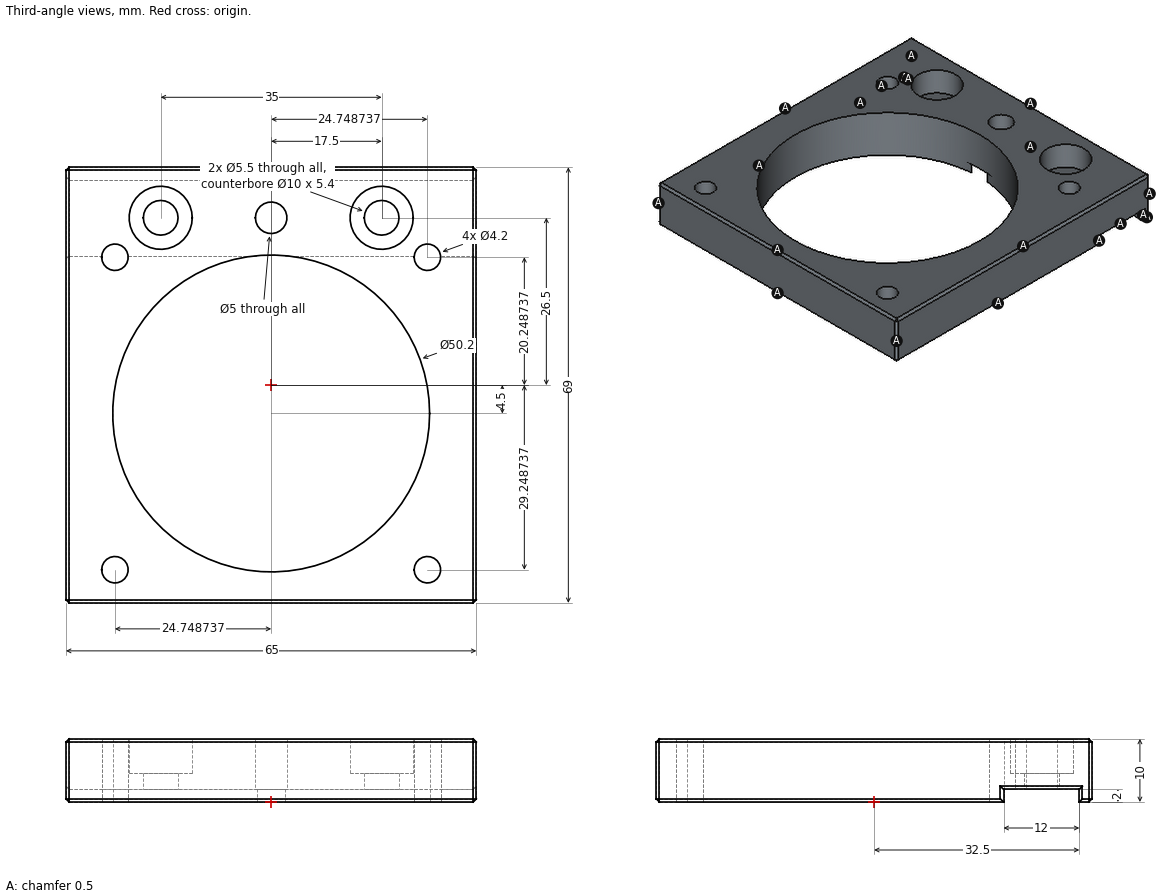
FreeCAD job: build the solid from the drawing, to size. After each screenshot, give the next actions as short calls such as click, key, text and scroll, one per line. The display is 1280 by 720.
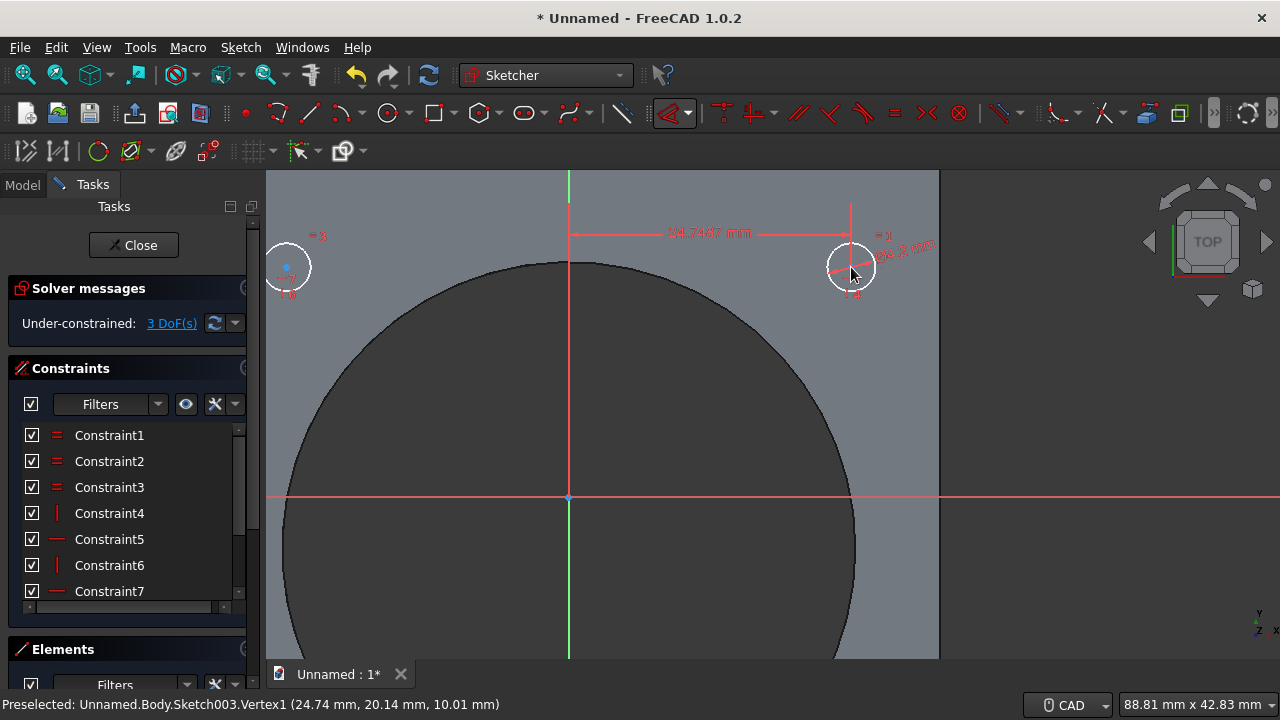
click(851, 267)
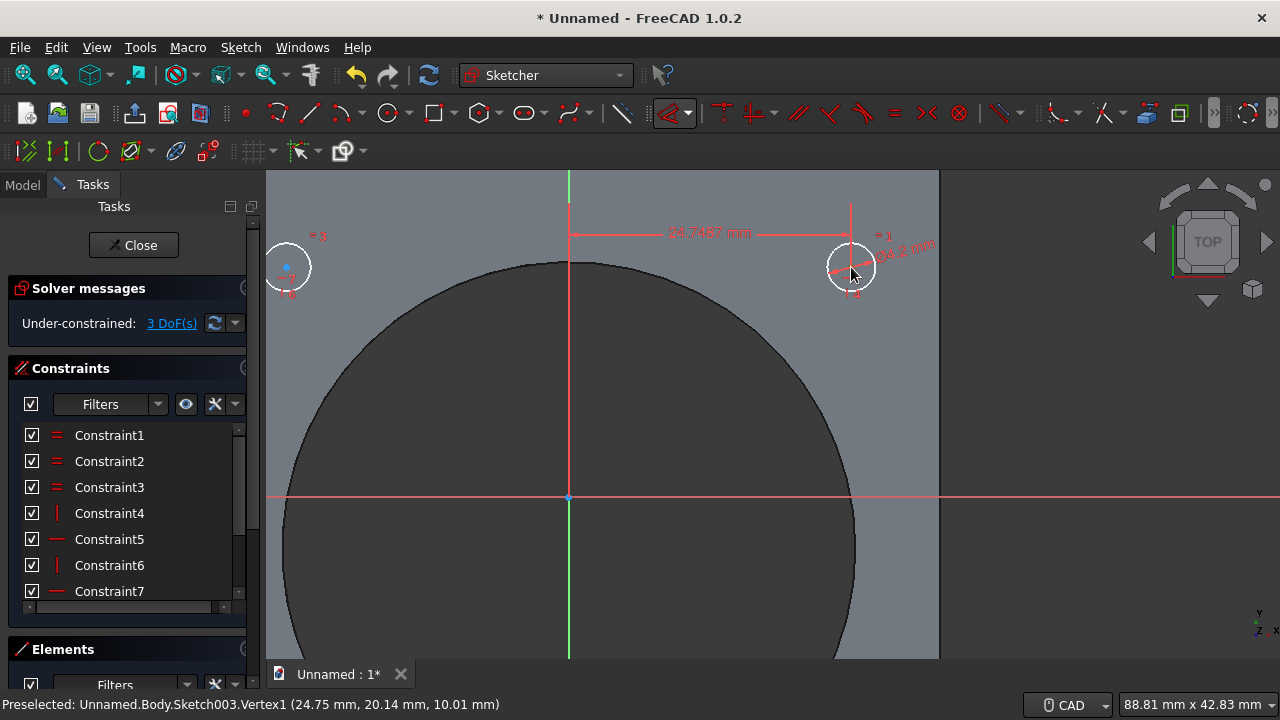
click(690, 114)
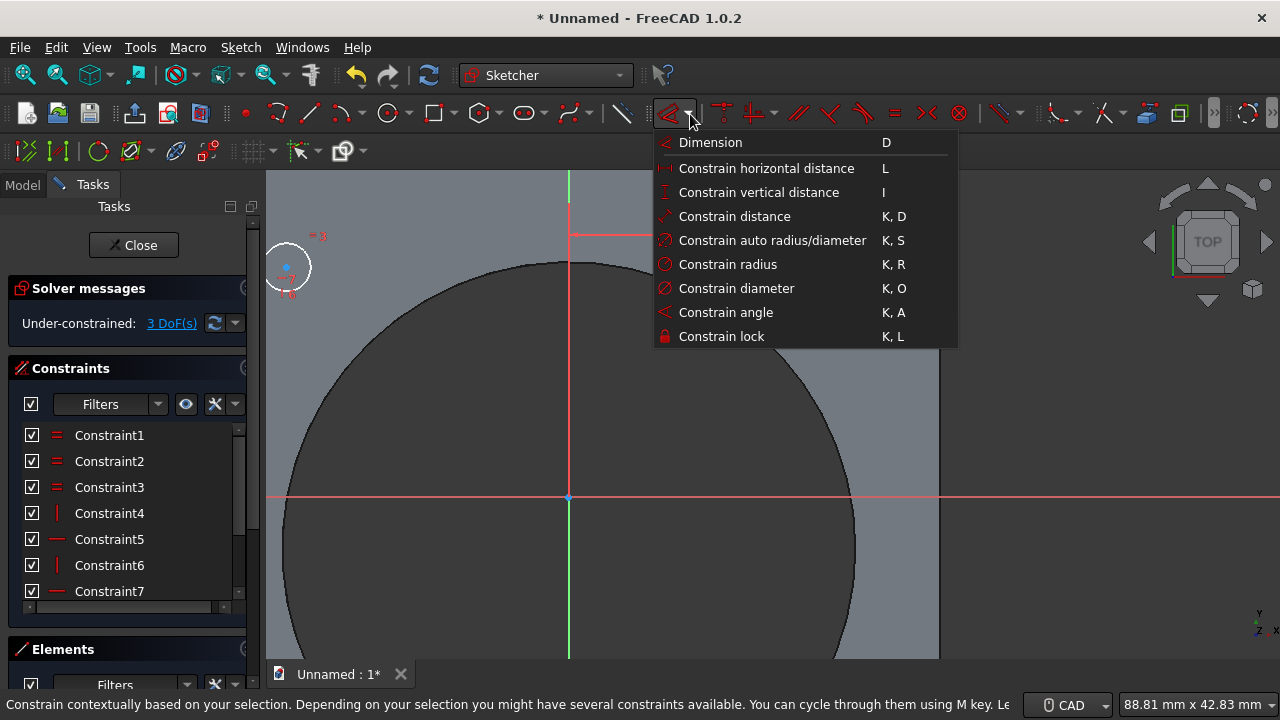
click(806, 192)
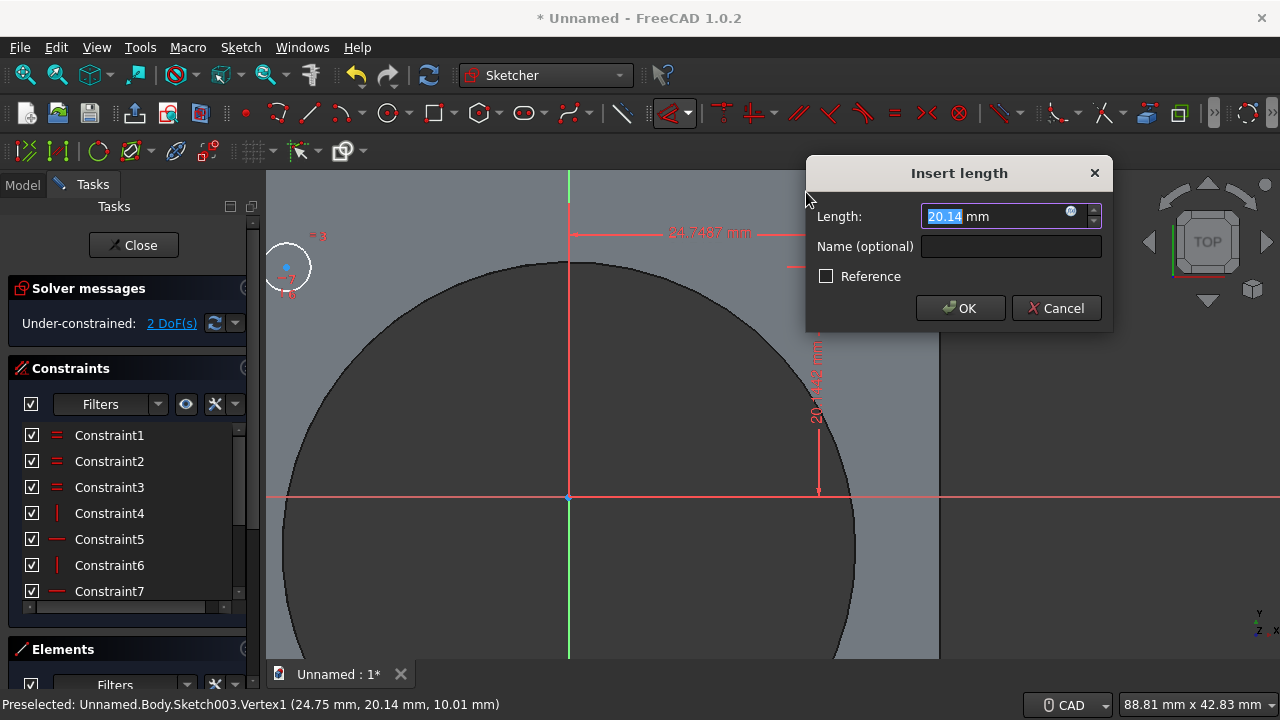
text(20.248737)
key(Return)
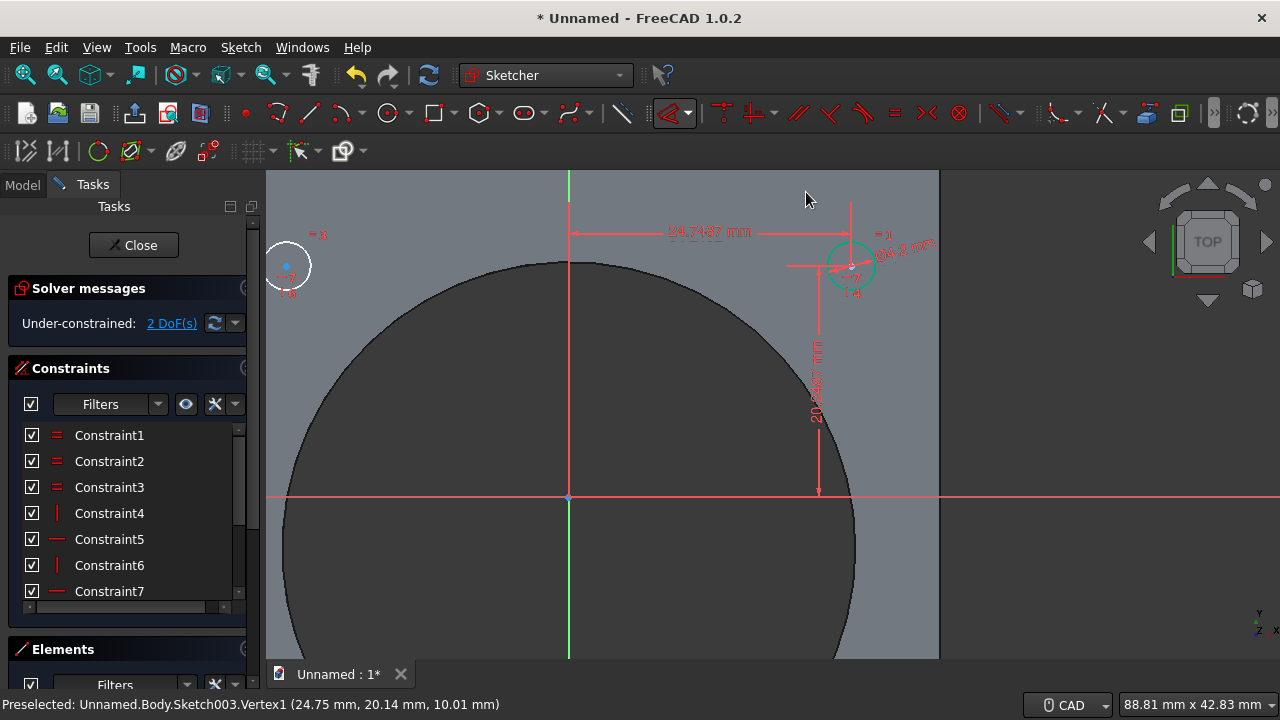
scroll(869, 251, down, 3)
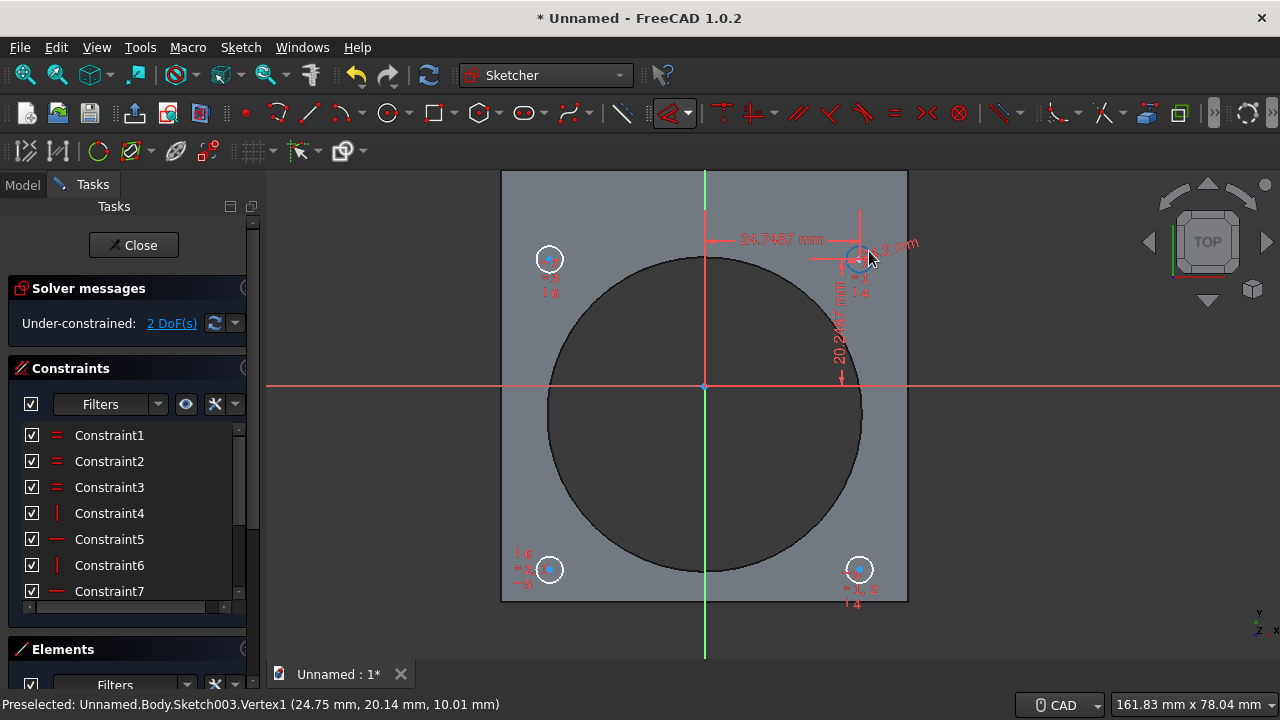
click(860, 570)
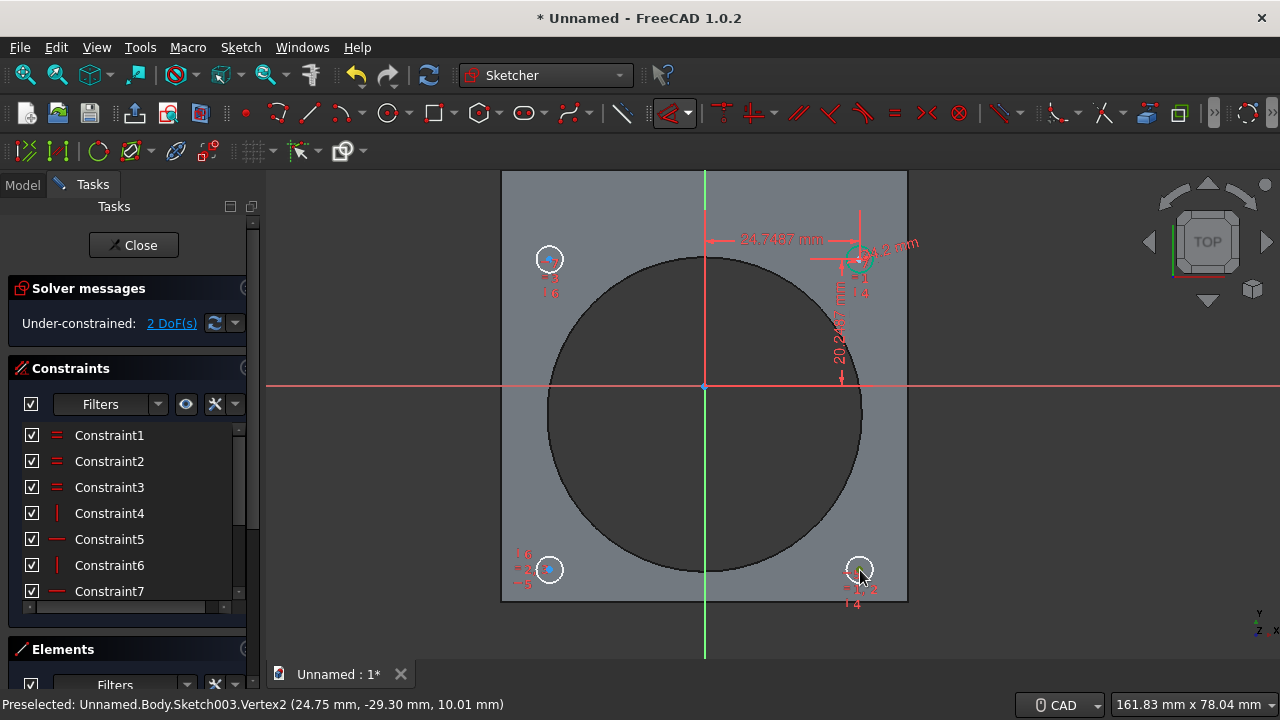
click(690, 114)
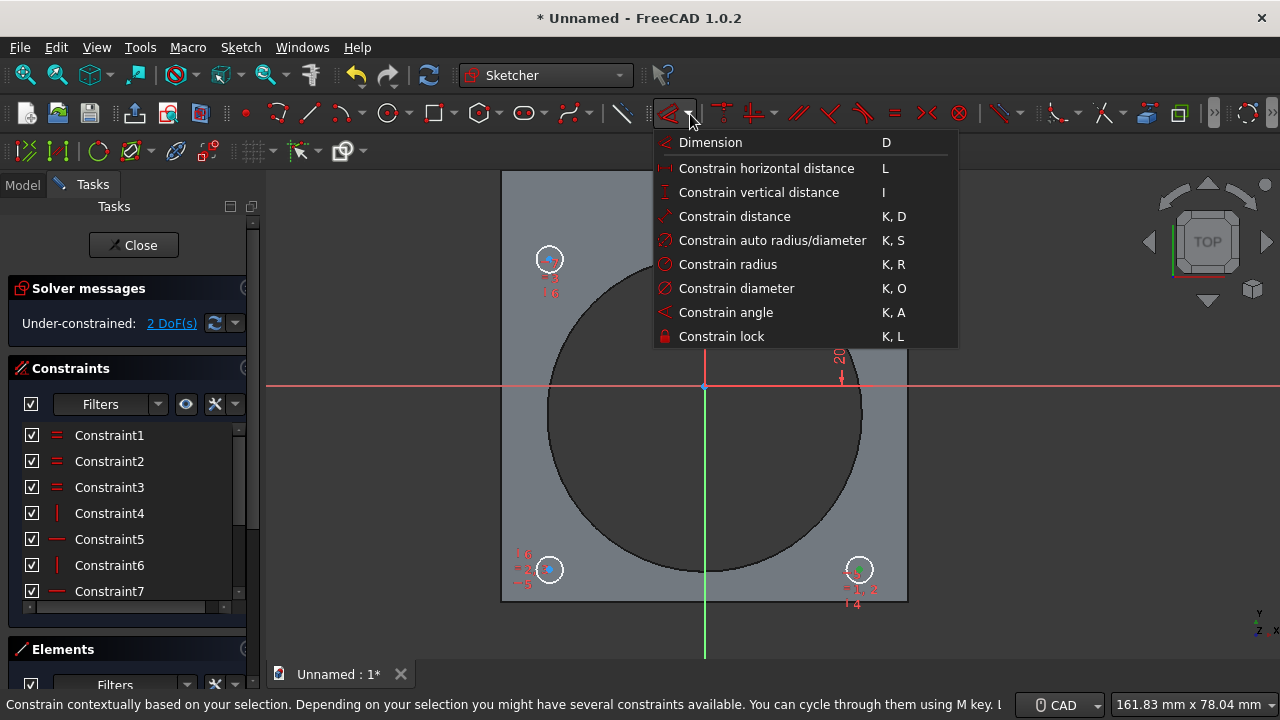
click(806, 192)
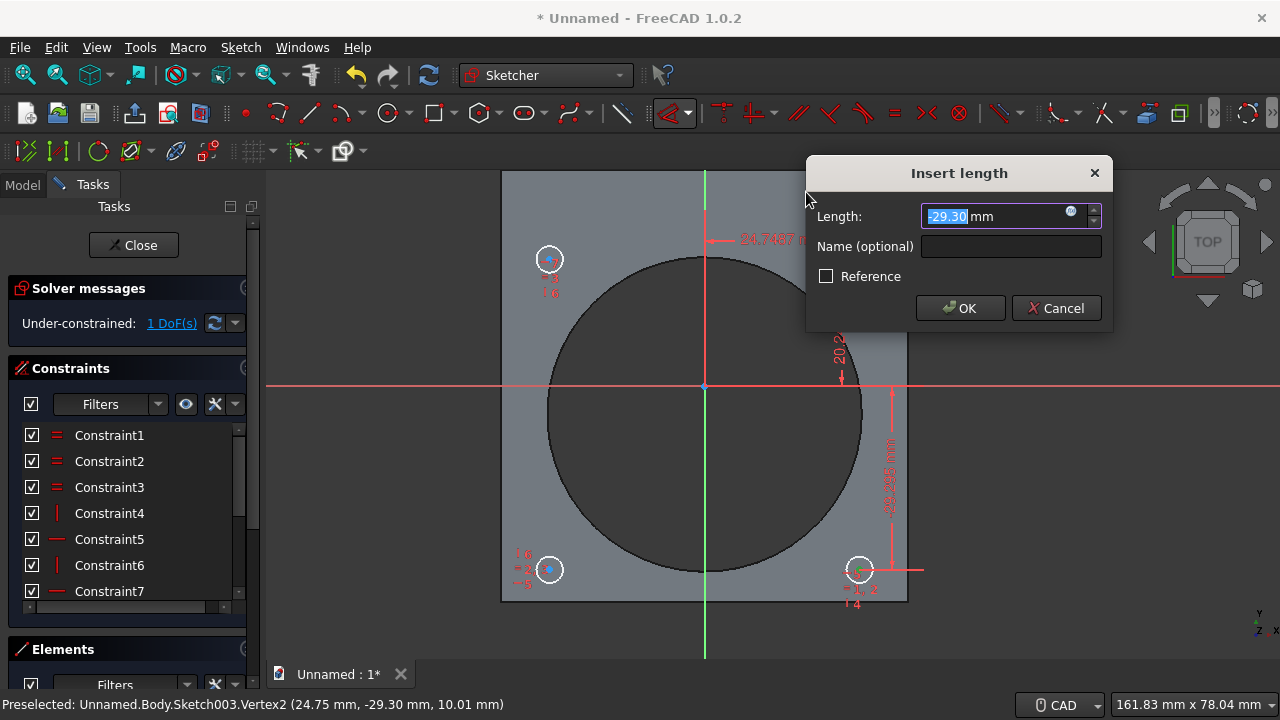
text(-29.248737)
key(Return)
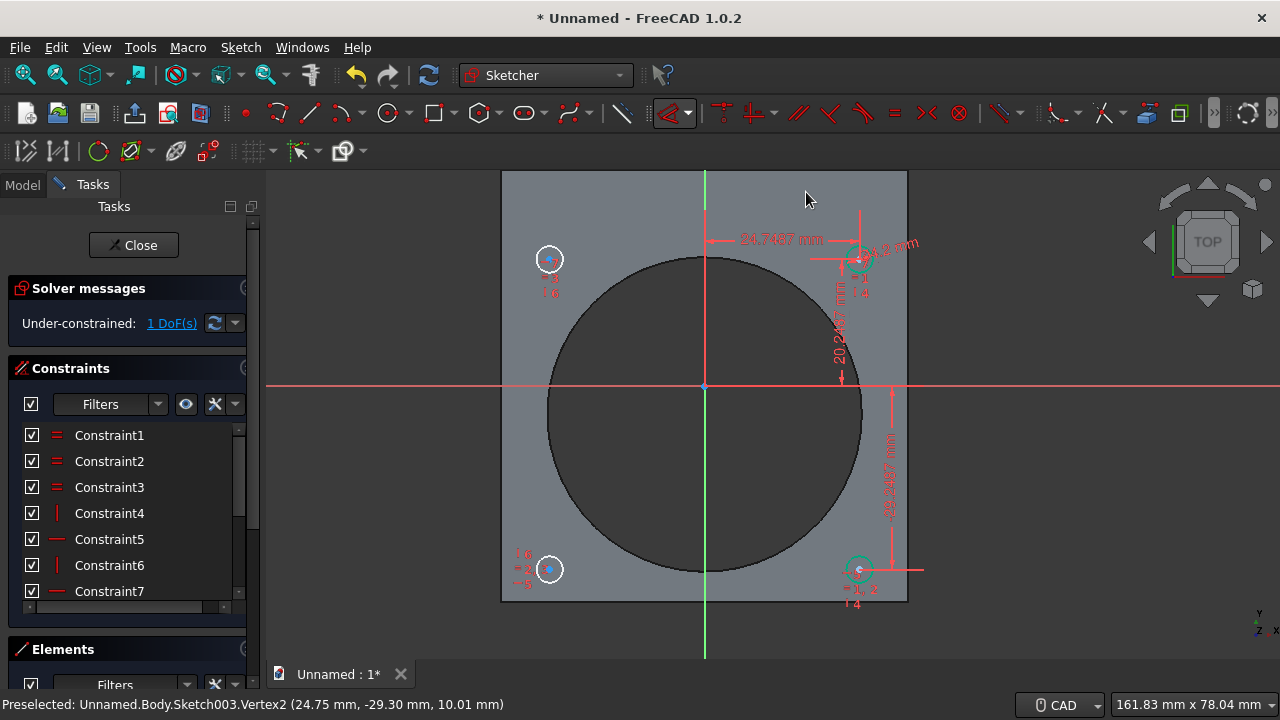
click(550, 570)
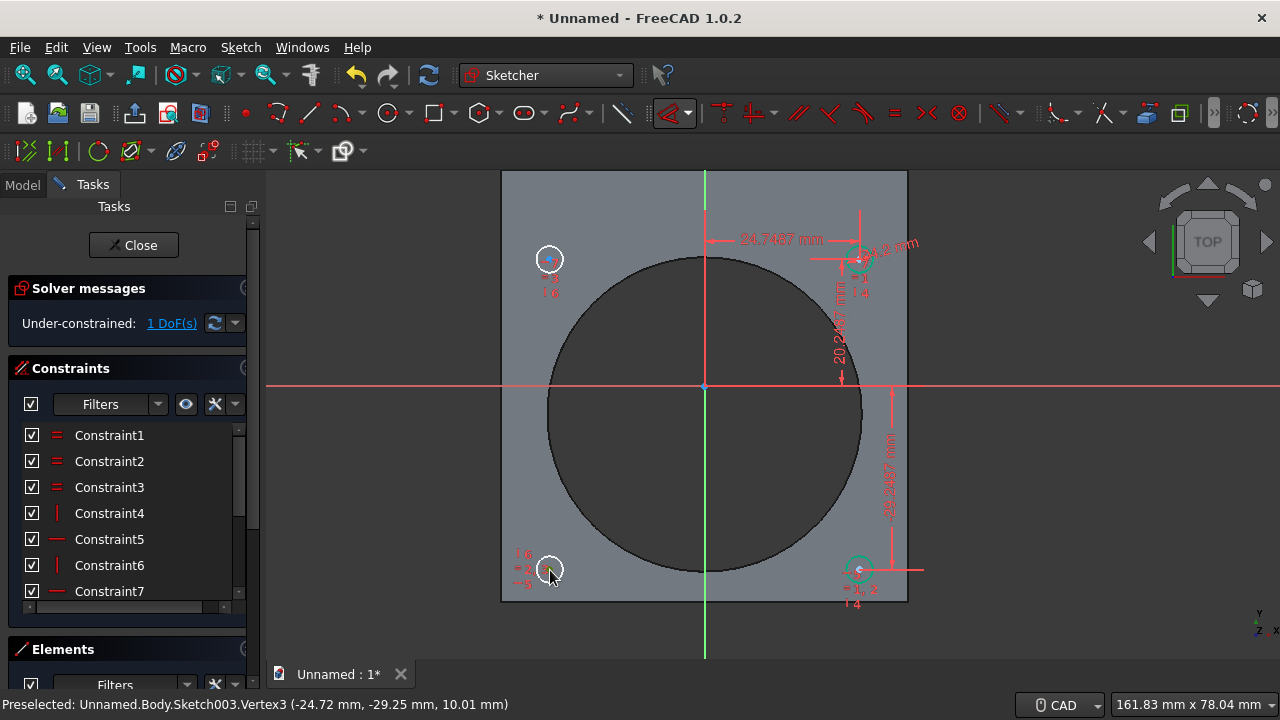
click(690, 114)